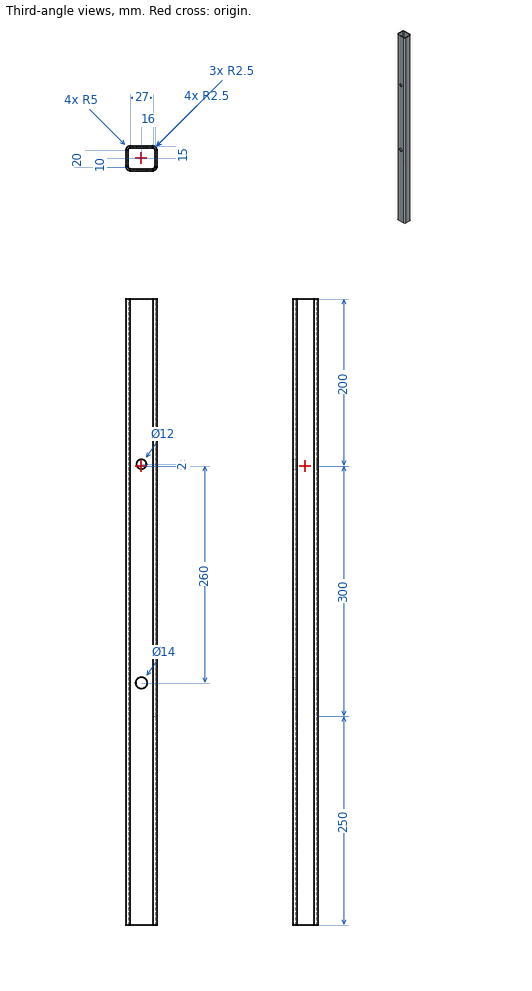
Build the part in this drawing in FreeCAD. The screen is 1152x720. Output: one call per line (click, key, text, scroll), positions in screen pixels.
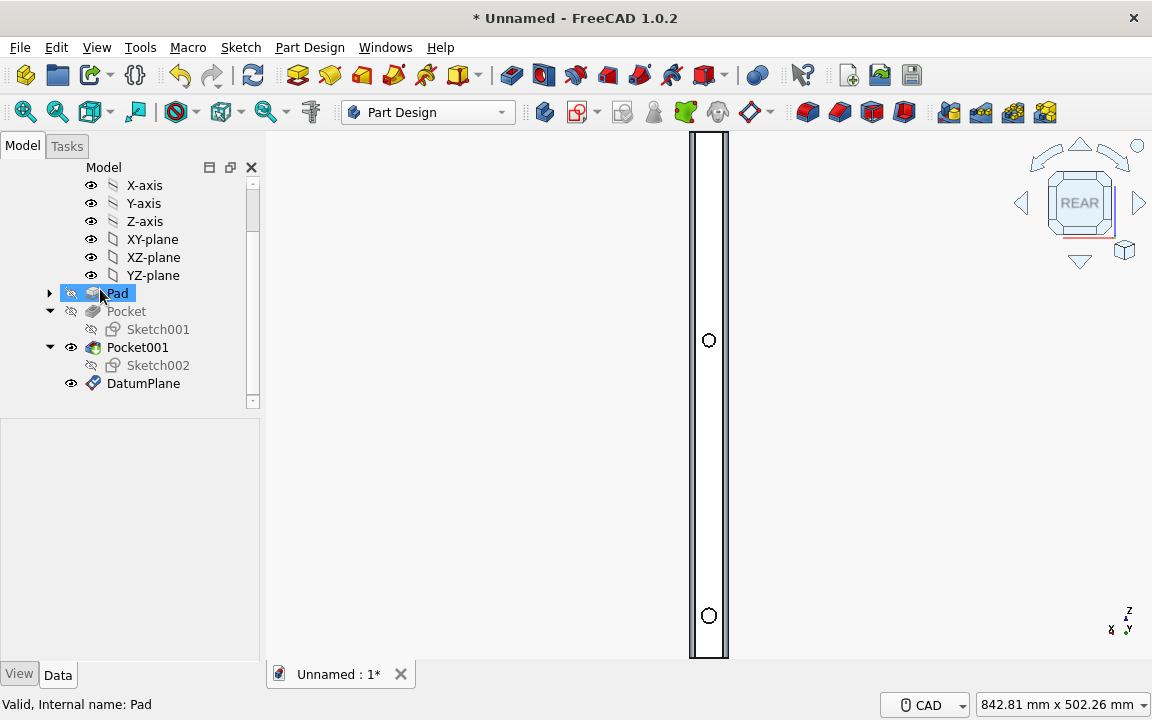
click(116, 383)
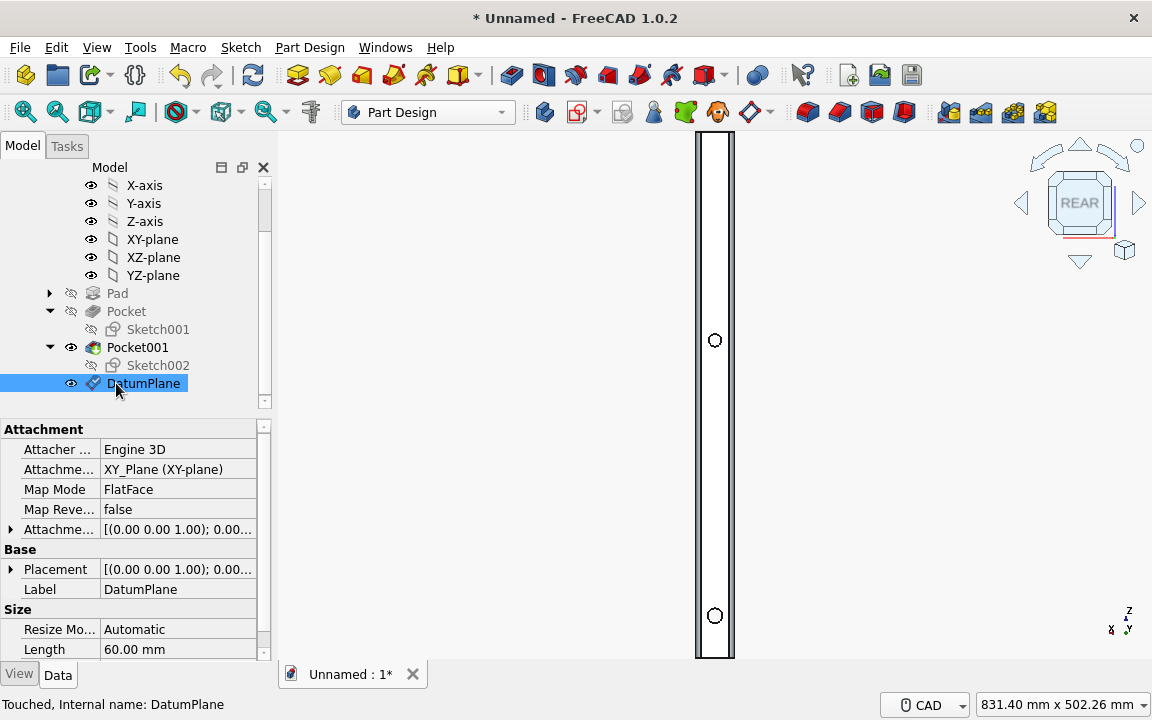
click(578, 112)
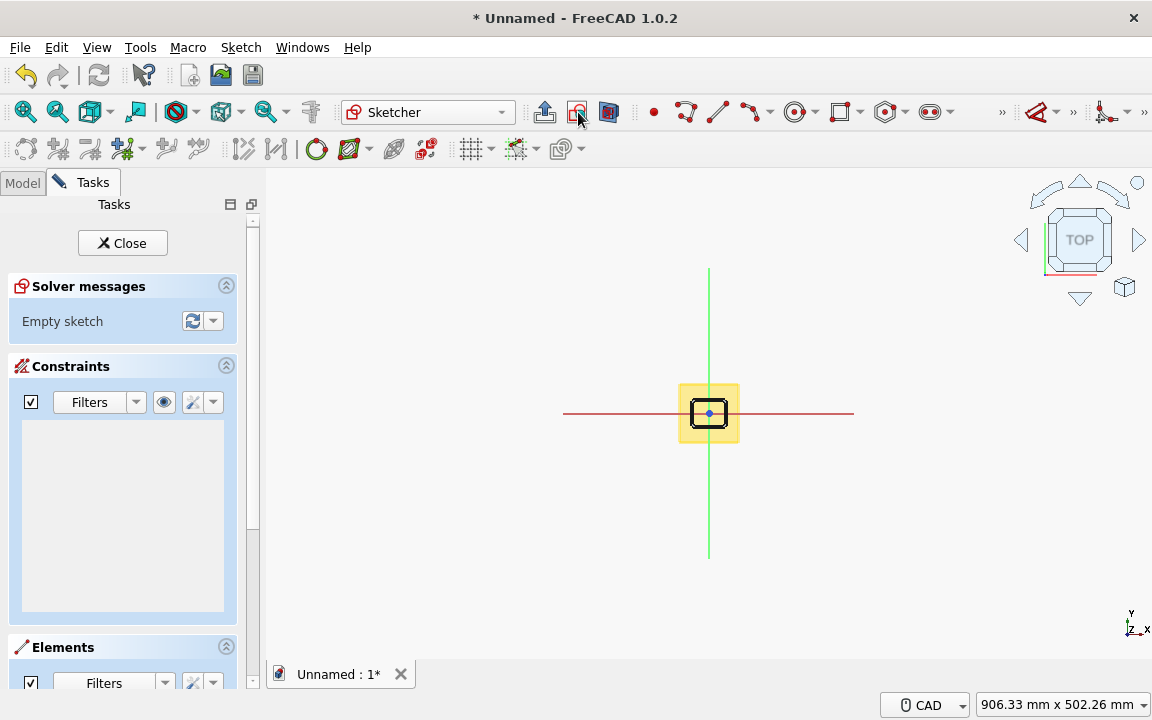
click(610, 112)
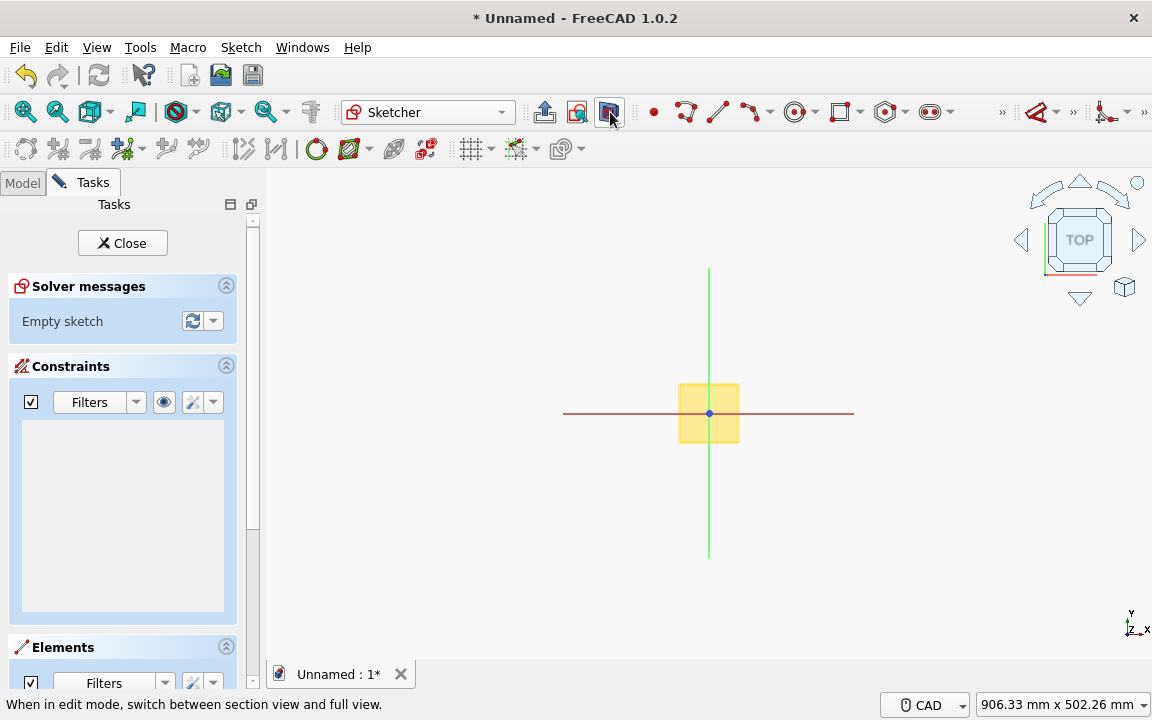
scroll(716, 413, up, 12)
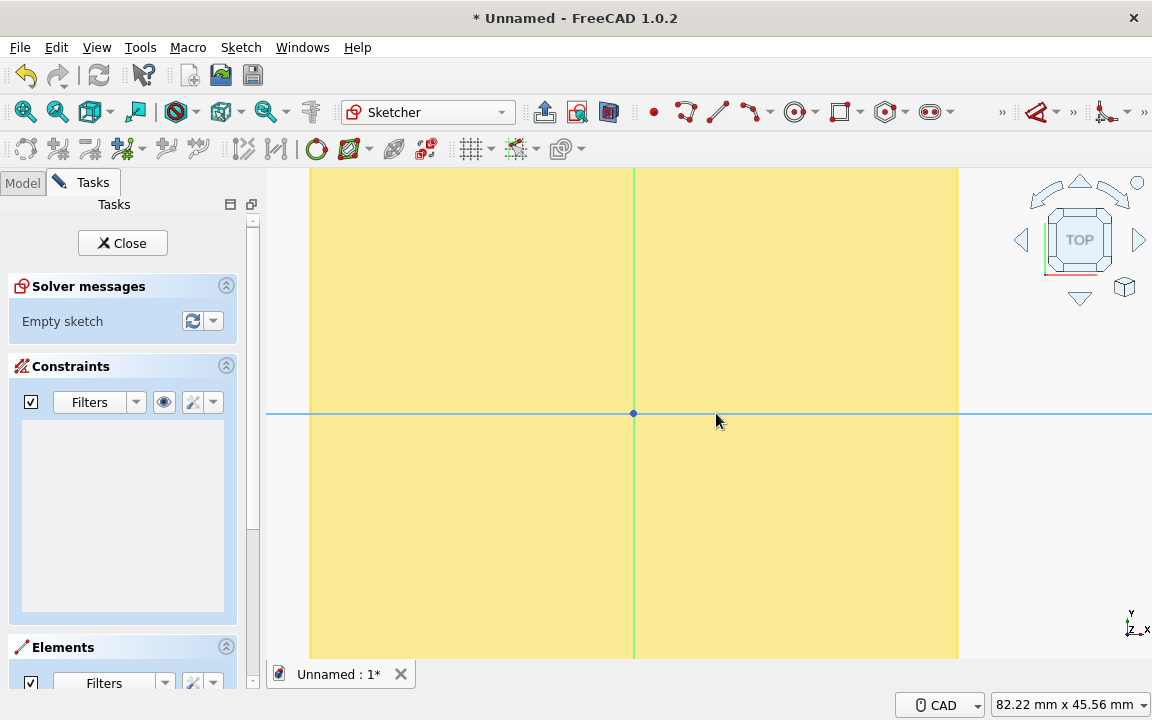
key(g)
key(l)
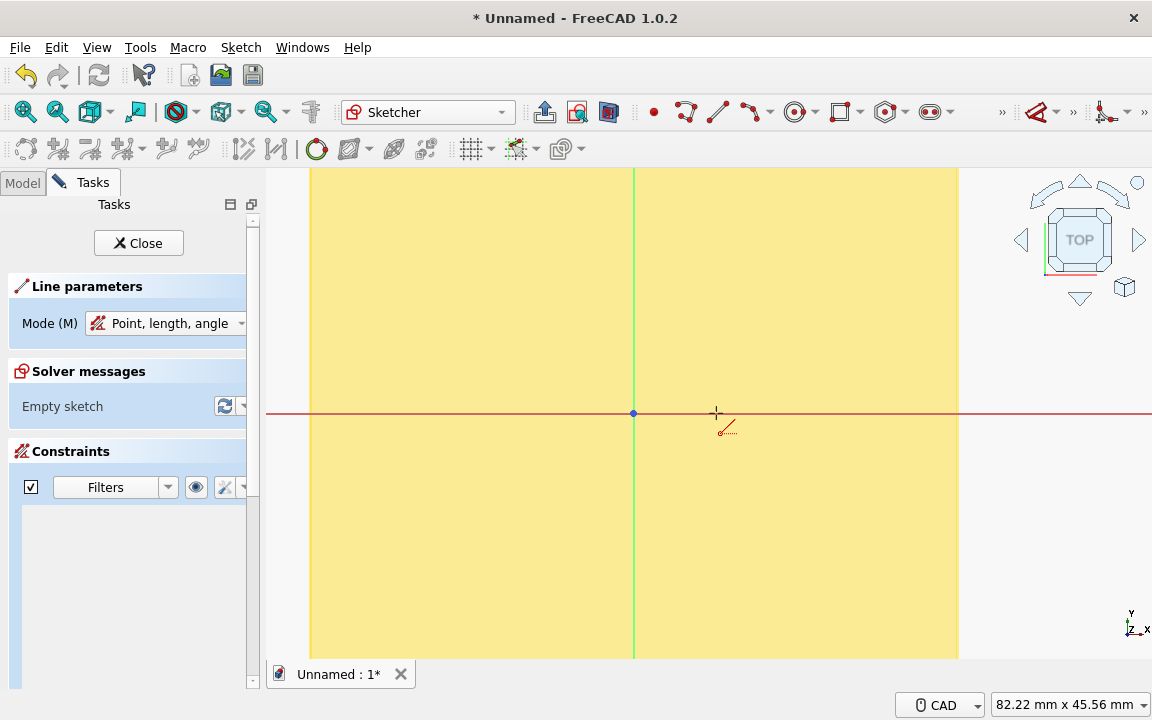
click(434, 521)
click(434, 306)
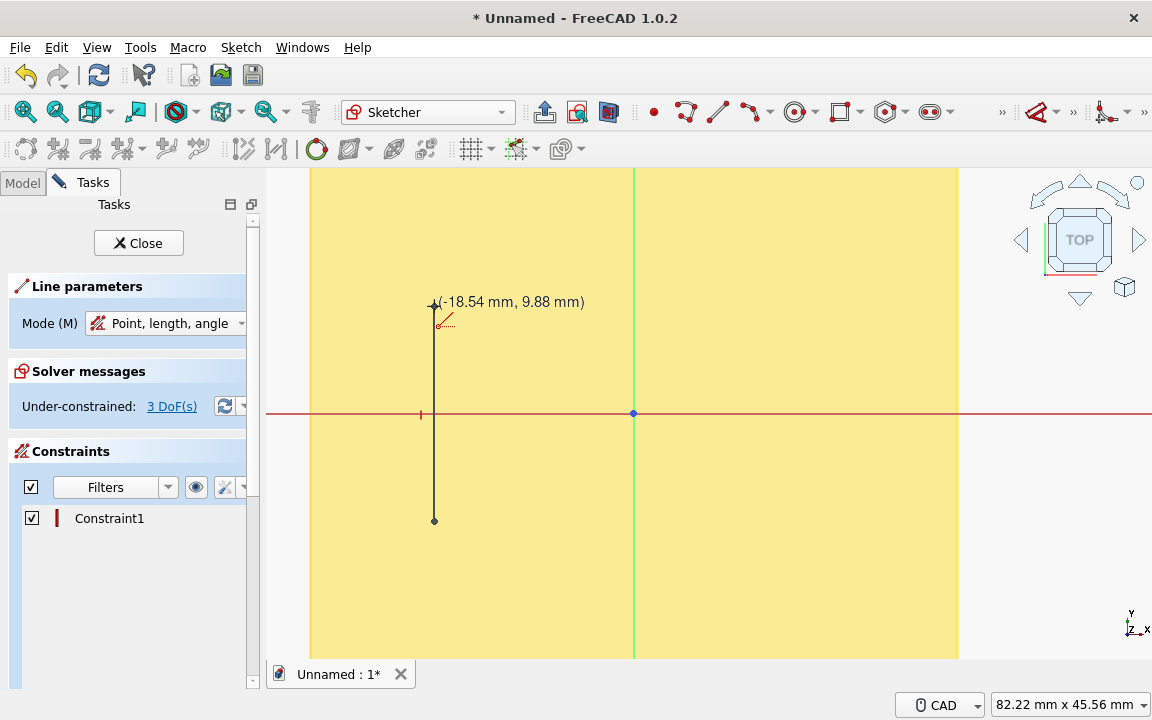
click(488, 252)
click(779, 252)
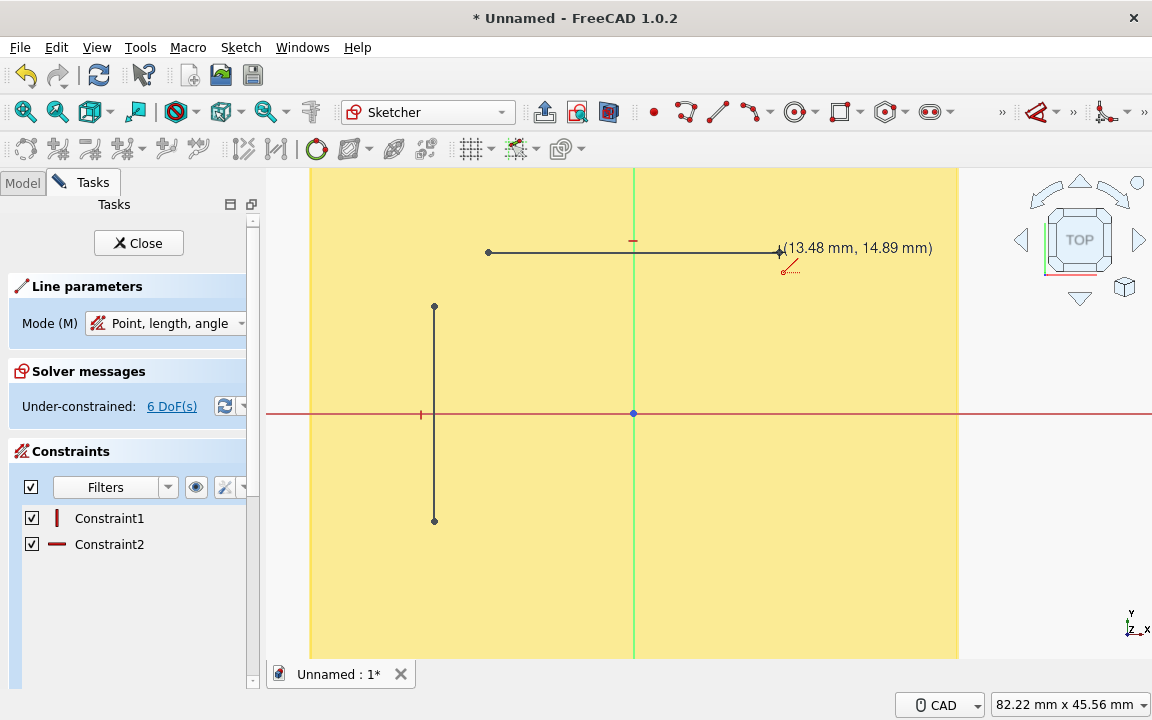
click(833, 306)
click(833, 521)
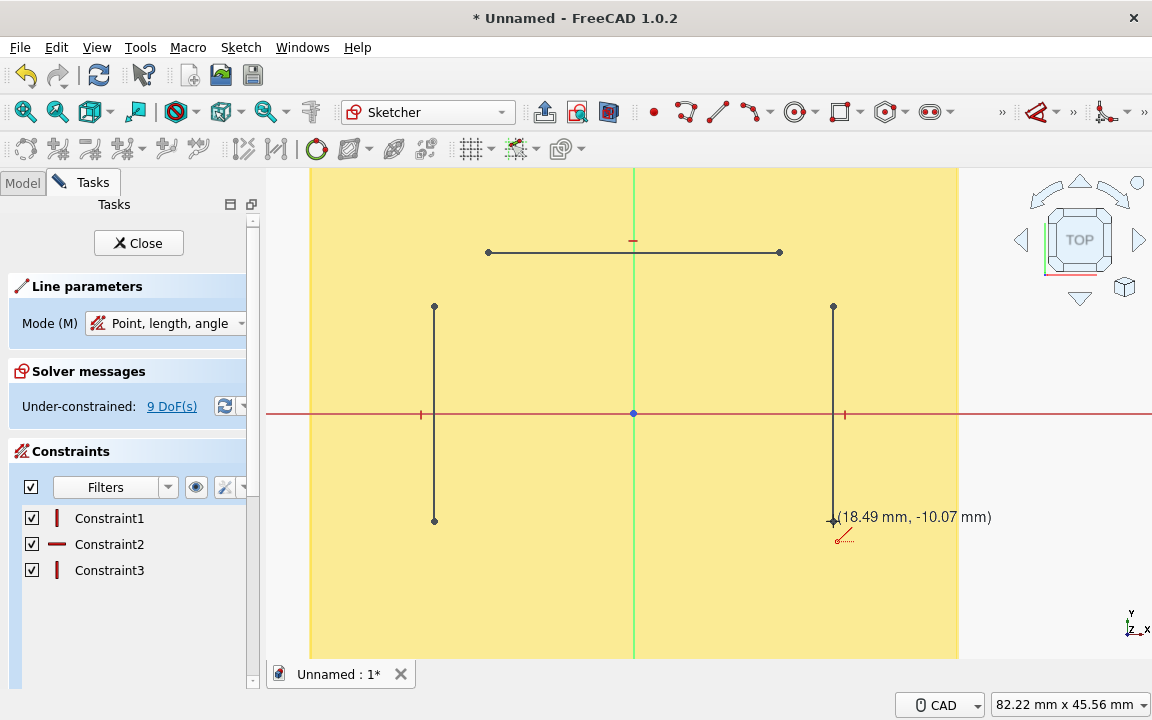
click(779, 575)
click(488, 575)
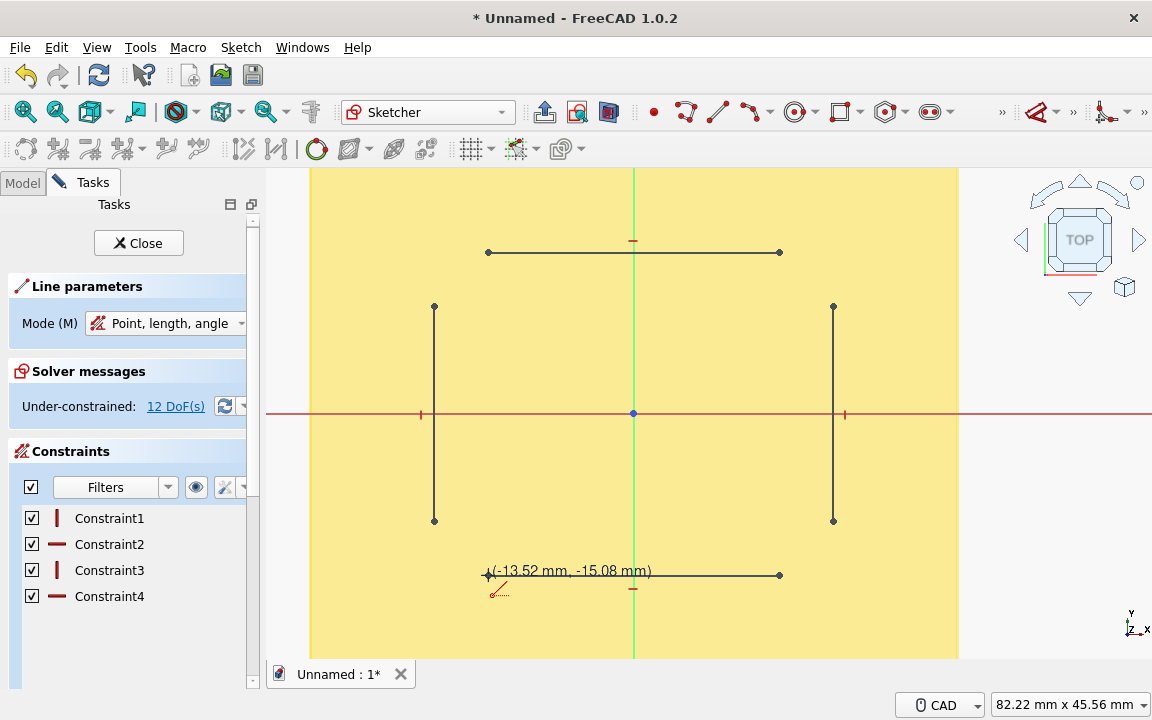
click(750, 112)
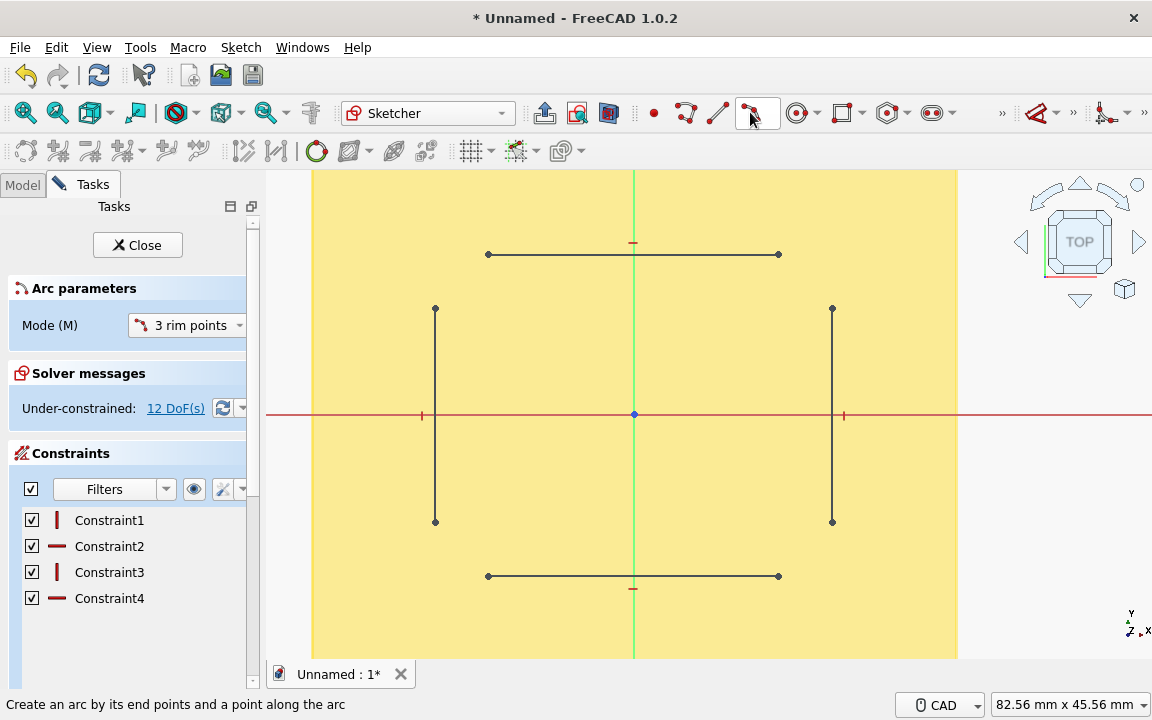
click(435, 308)
click(489, 255)
click(451, 269)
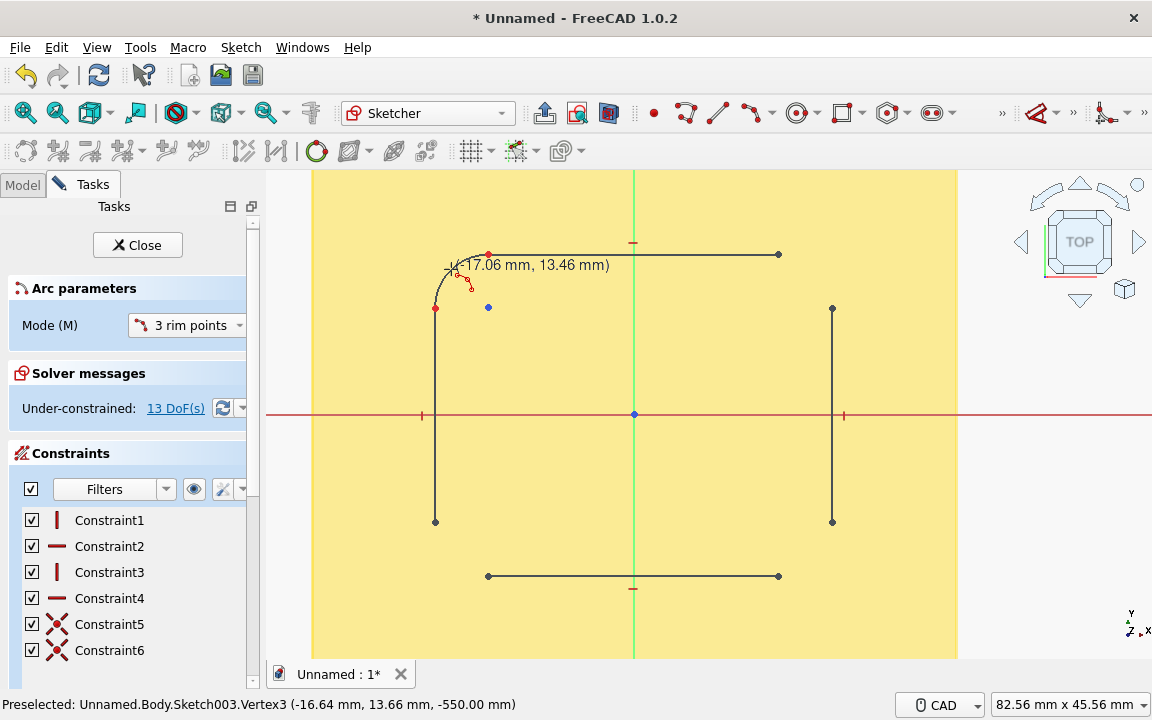
click(779, 255)
click(832, 308)
click(817, 269)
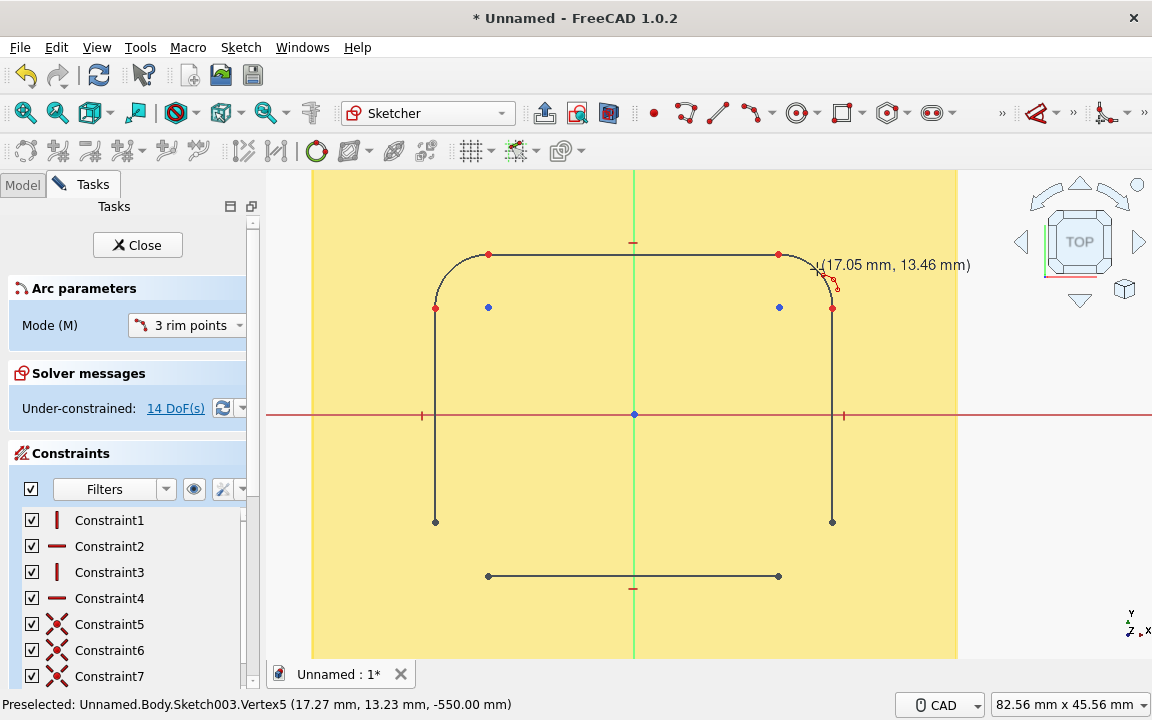
click(832, 523)
click(779, 576)
click(817, 560)